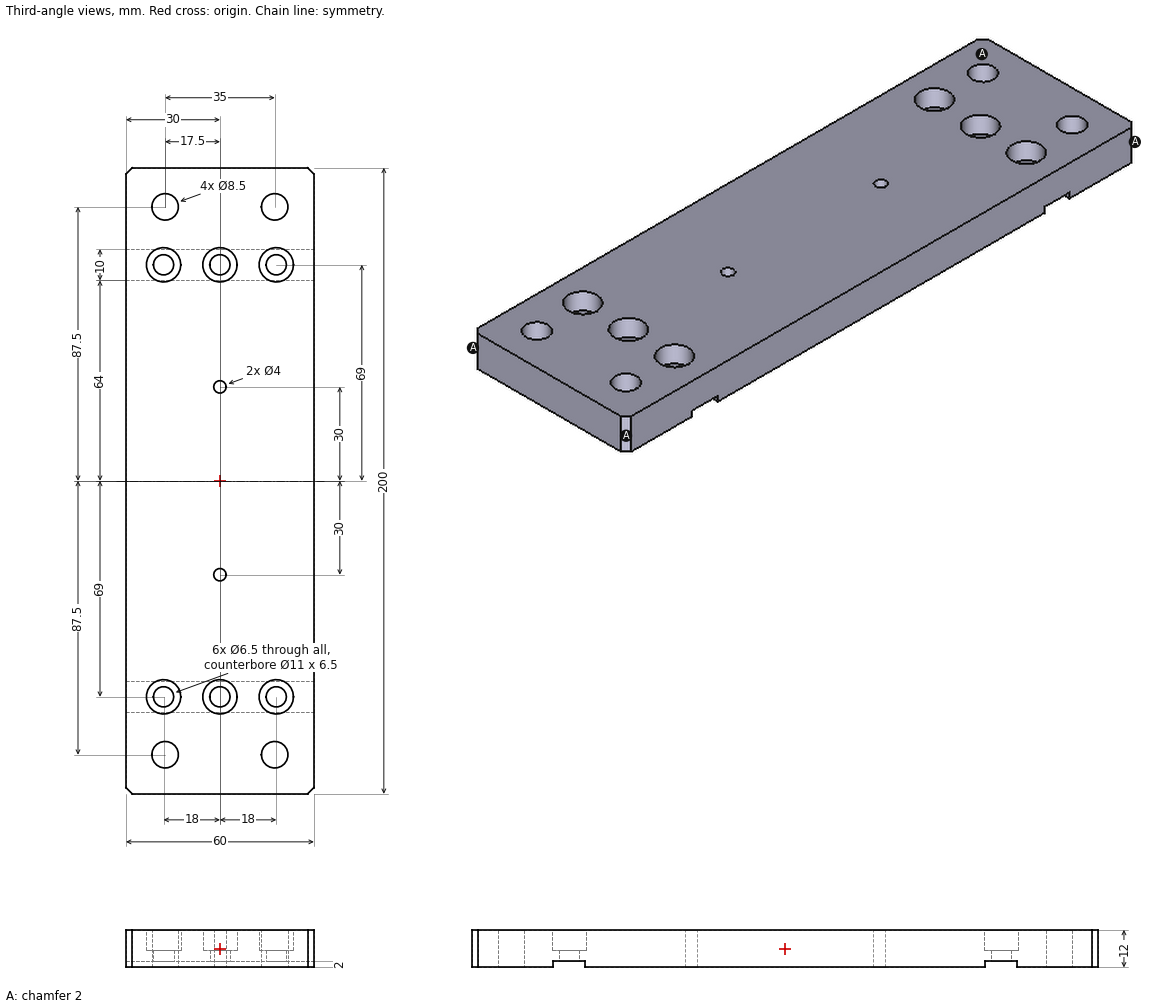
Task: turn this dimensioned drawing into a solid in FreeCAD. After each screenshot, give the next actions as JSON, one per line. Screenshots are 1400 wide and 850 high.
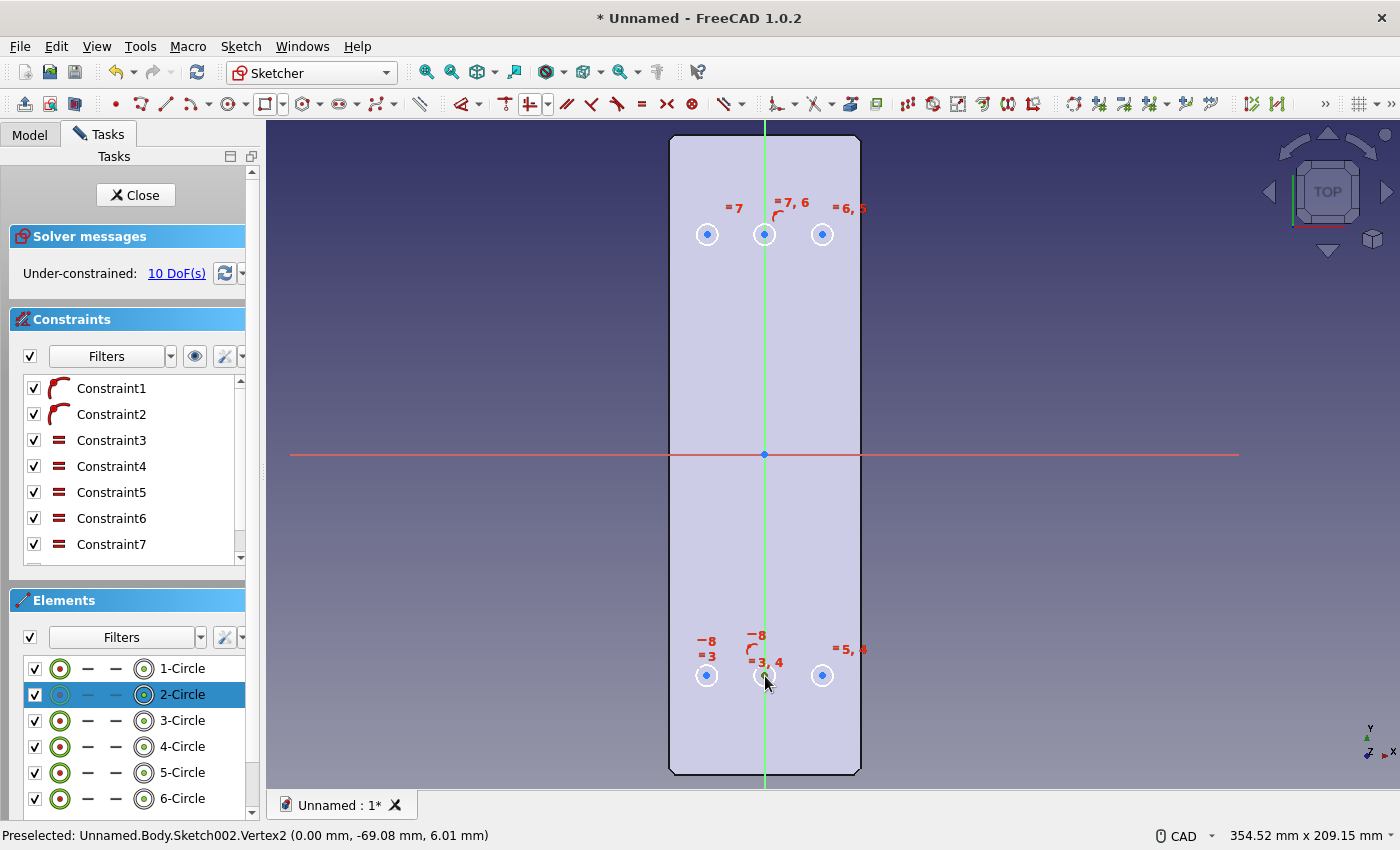
{"action": "left_click", "coordinate": [822, 676]}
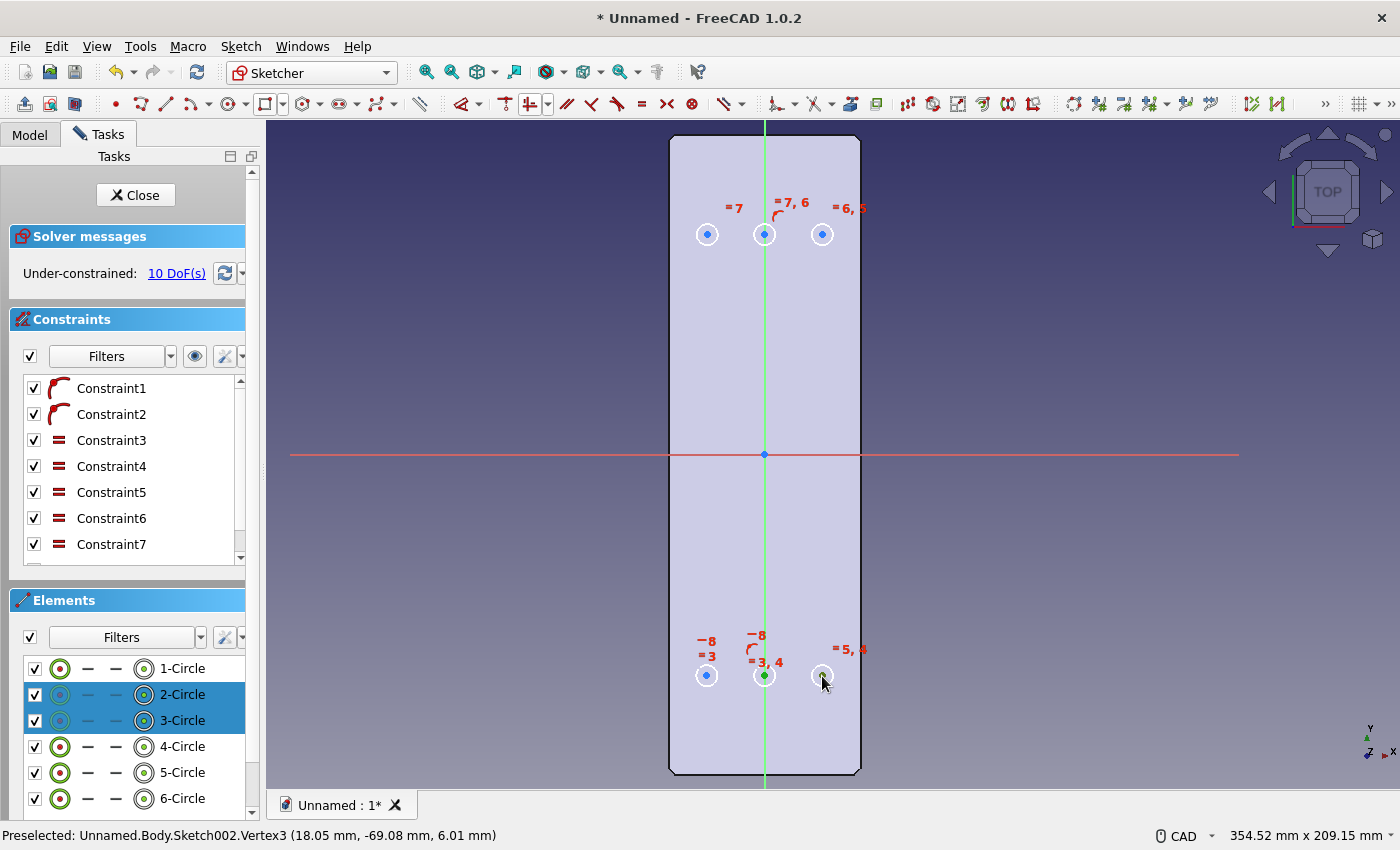
{"action": "key", "text": "h"}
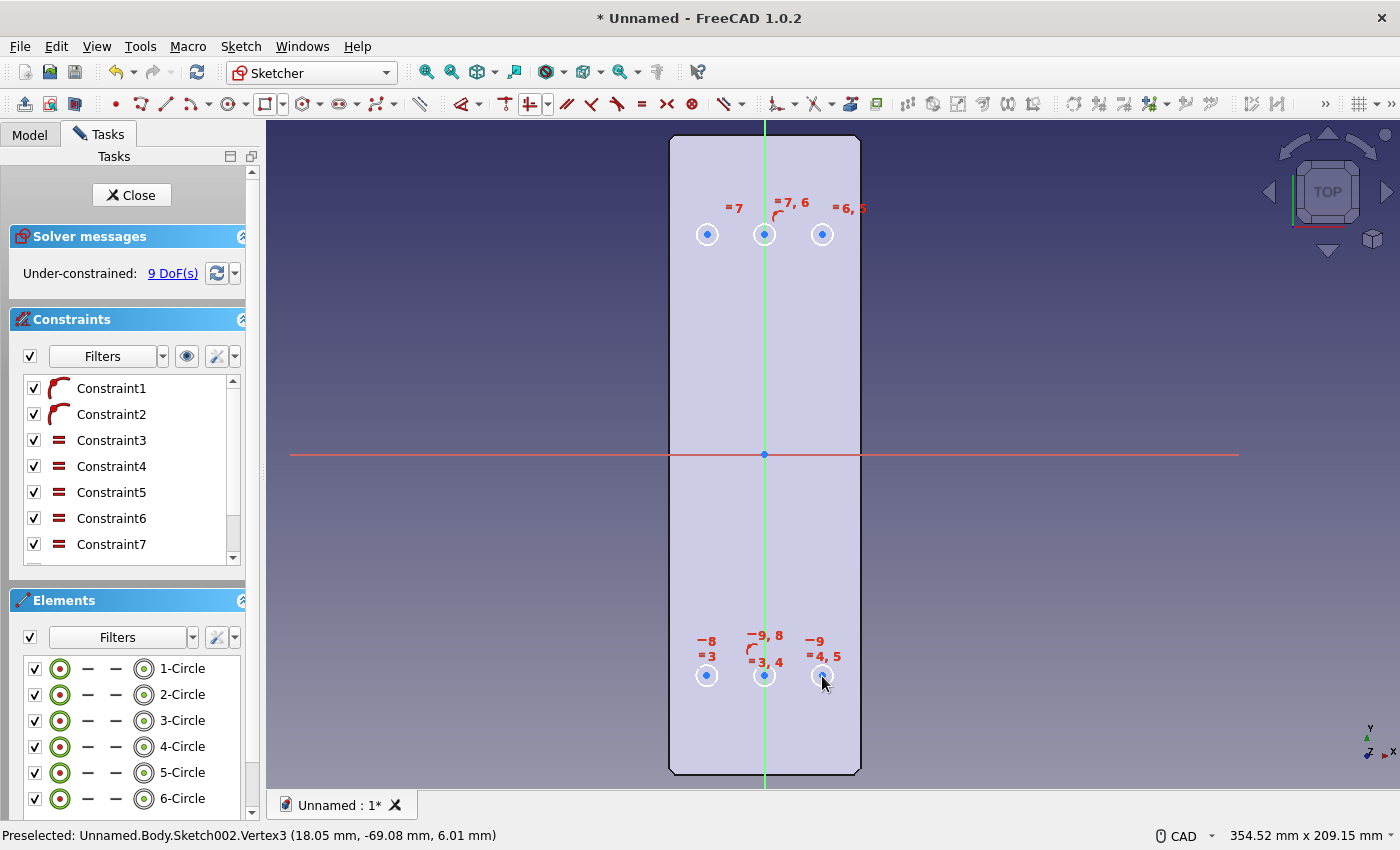
{"action": "left_click", "coordinate": [822, 676]}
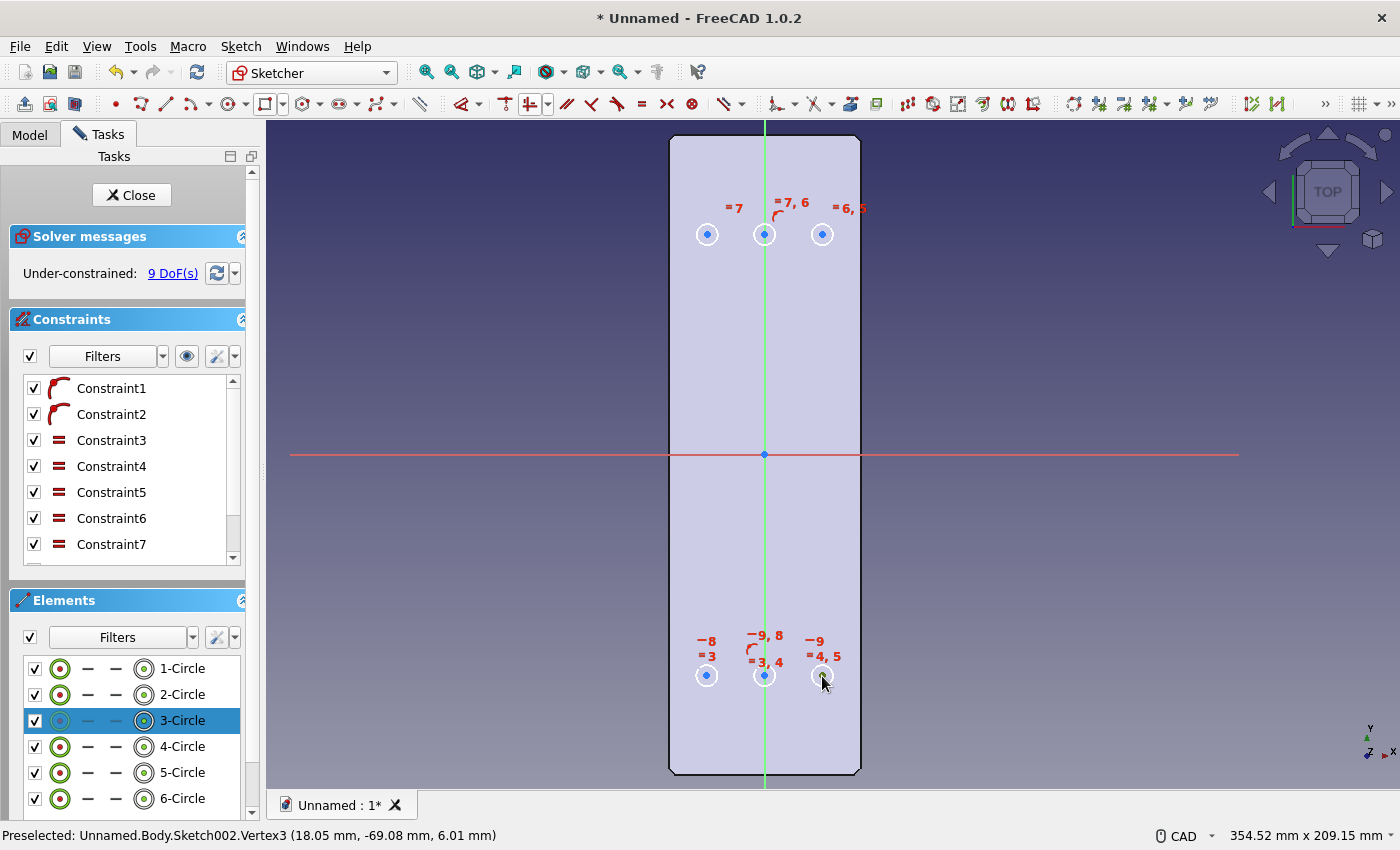
{"action": "left_click", "coordinate": [822, 235]}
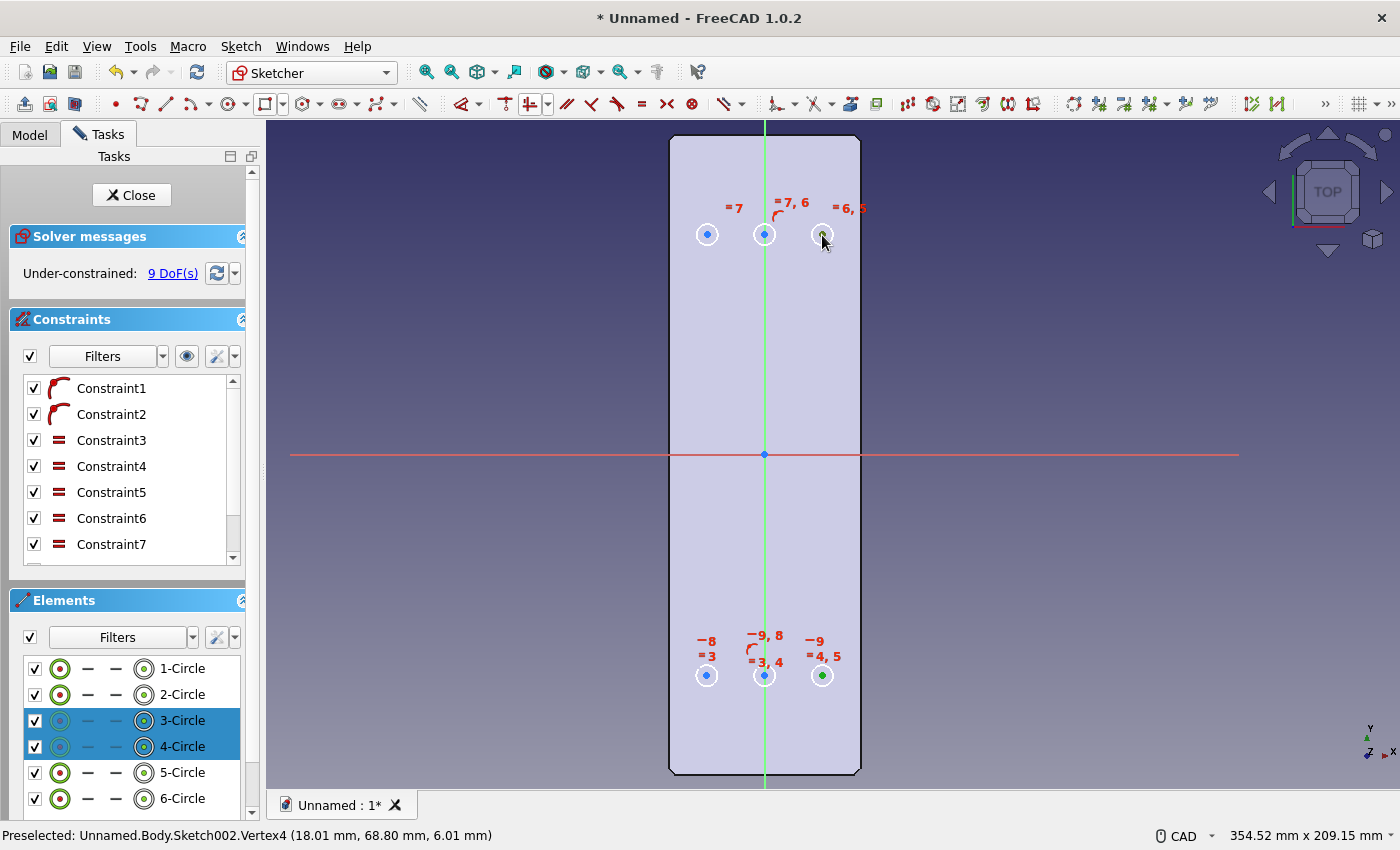
{"action": "key", "text": "v"}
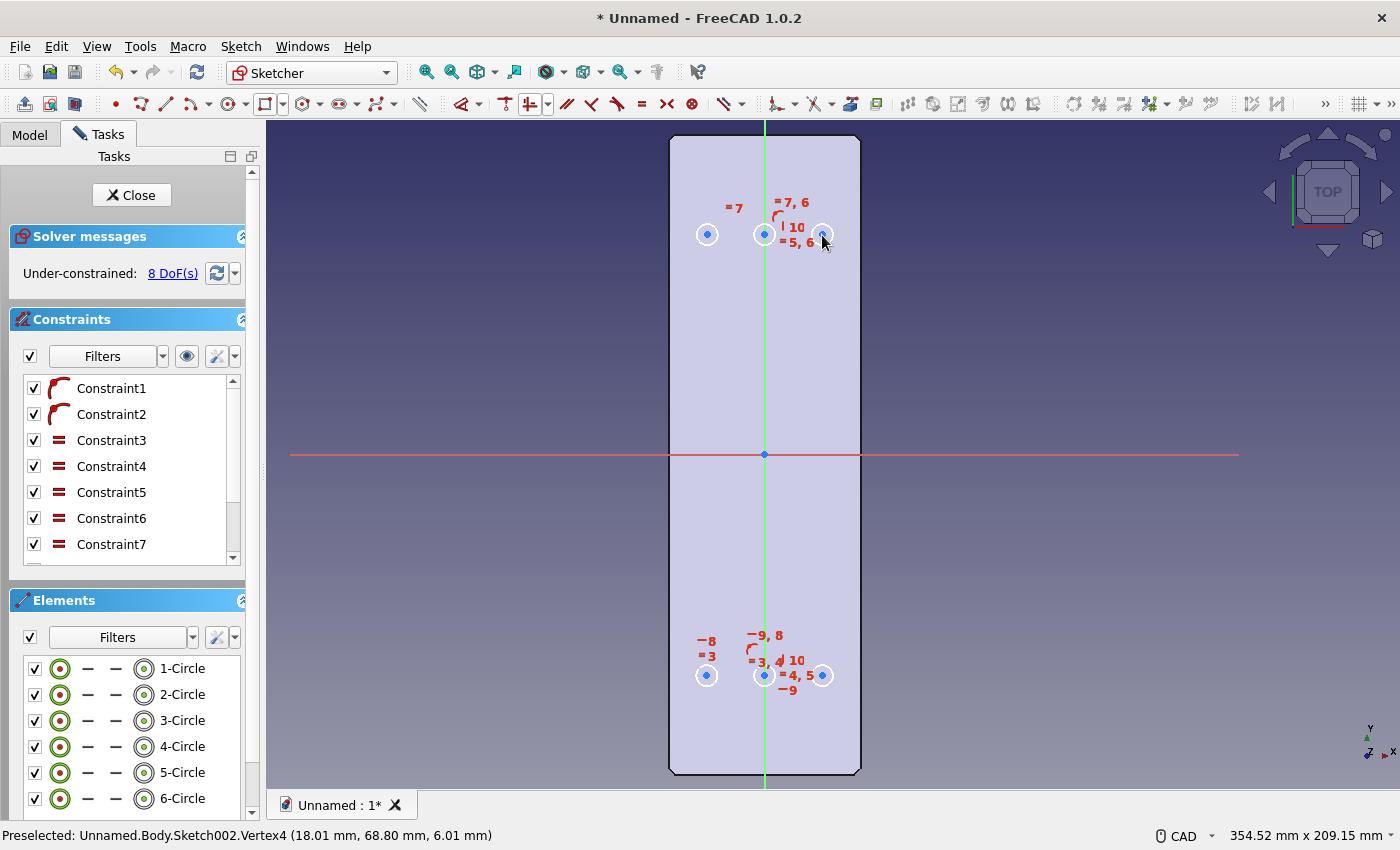
{"action": "left_click", "coordinate": [822, 235]}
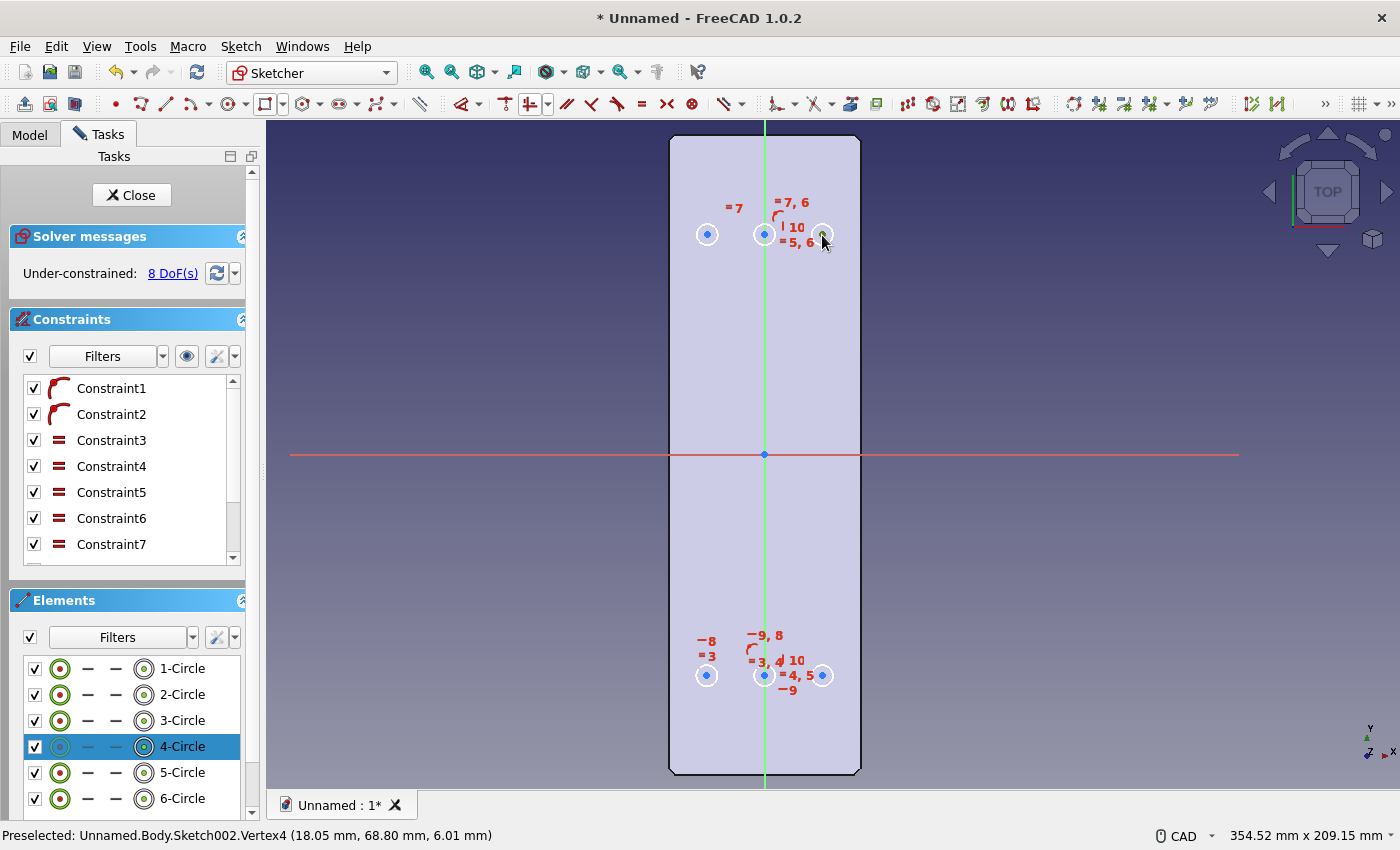
{"action": "left_click", "coordinate": [765, 235]}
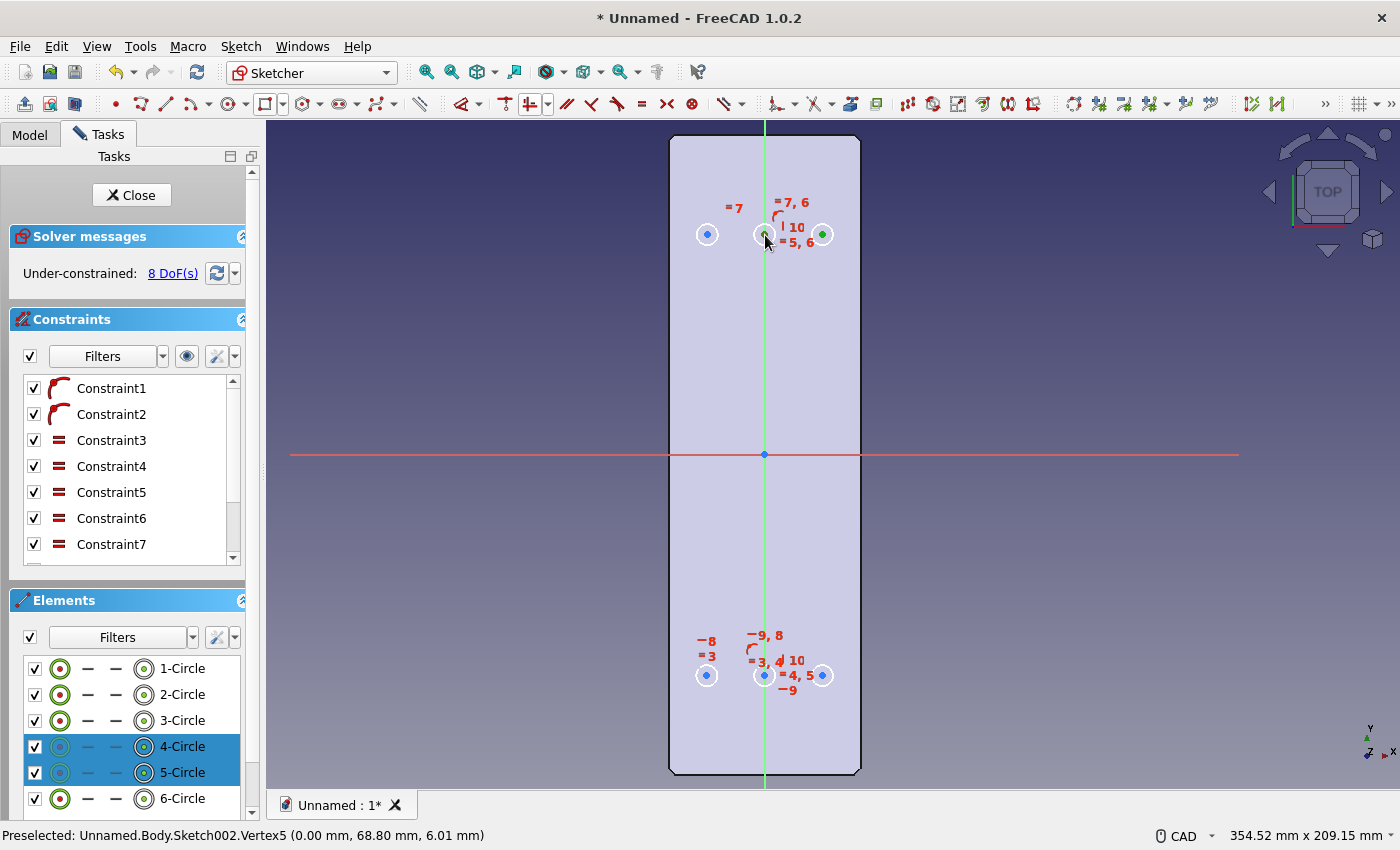
{"action": "left_click", "coordinate": [548, 104]}